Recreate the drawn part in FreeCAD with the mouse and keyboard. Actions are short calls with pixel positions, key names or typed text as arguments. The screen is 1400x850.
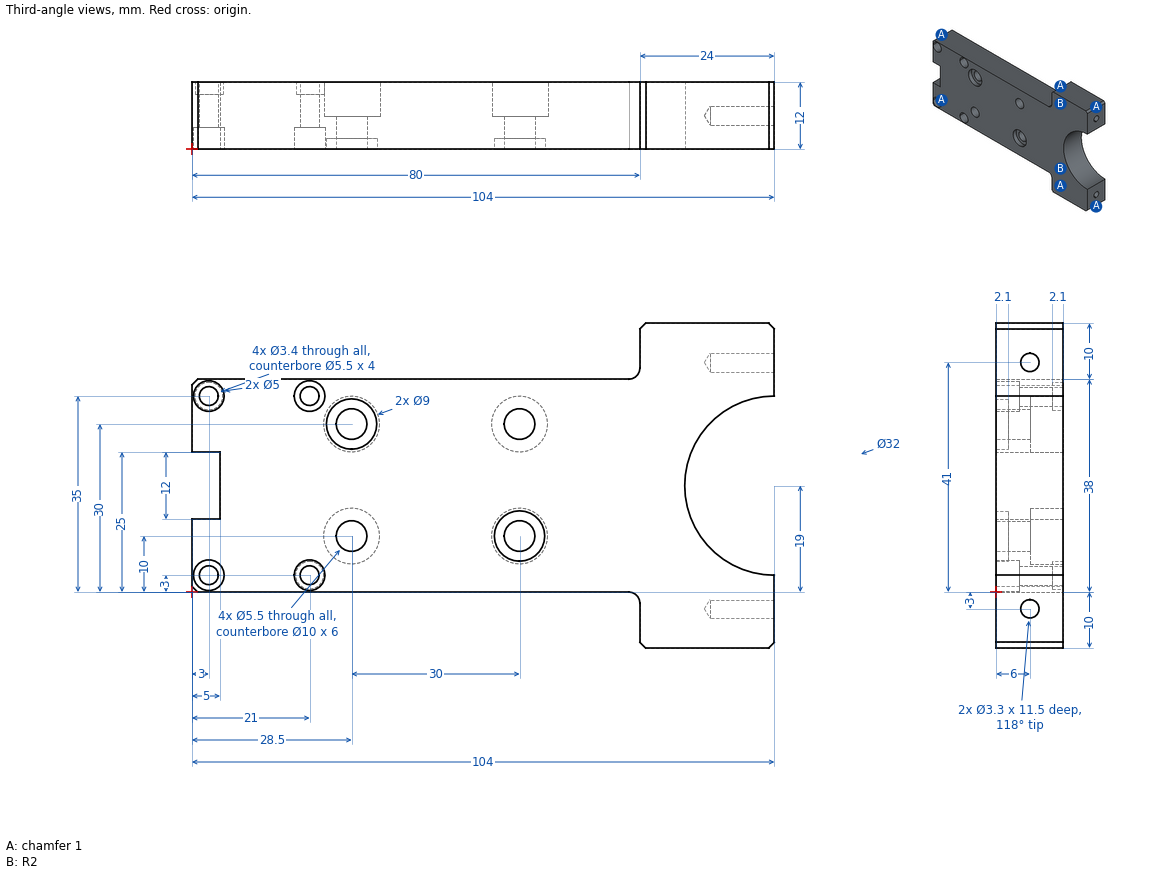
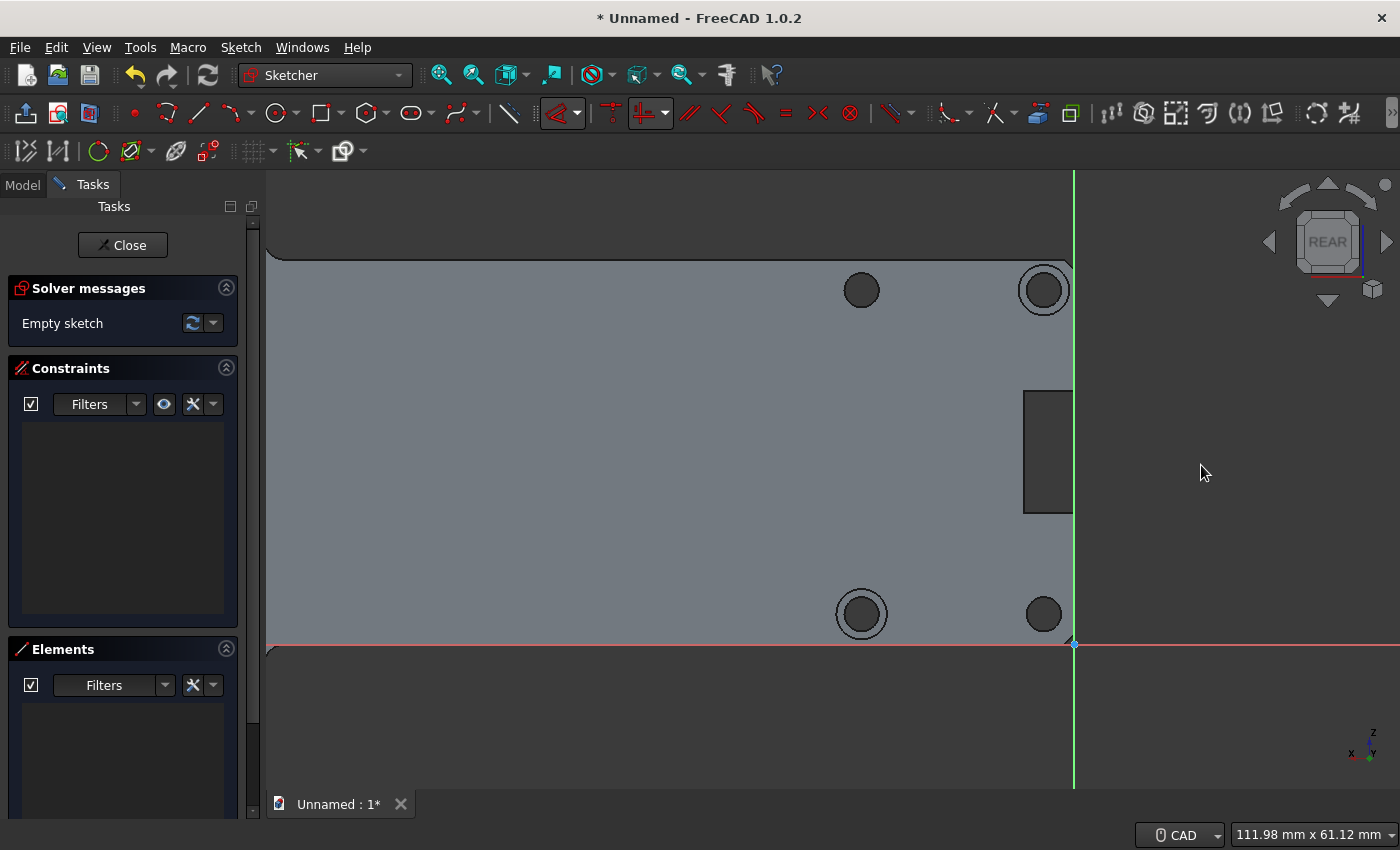
click(276, 114)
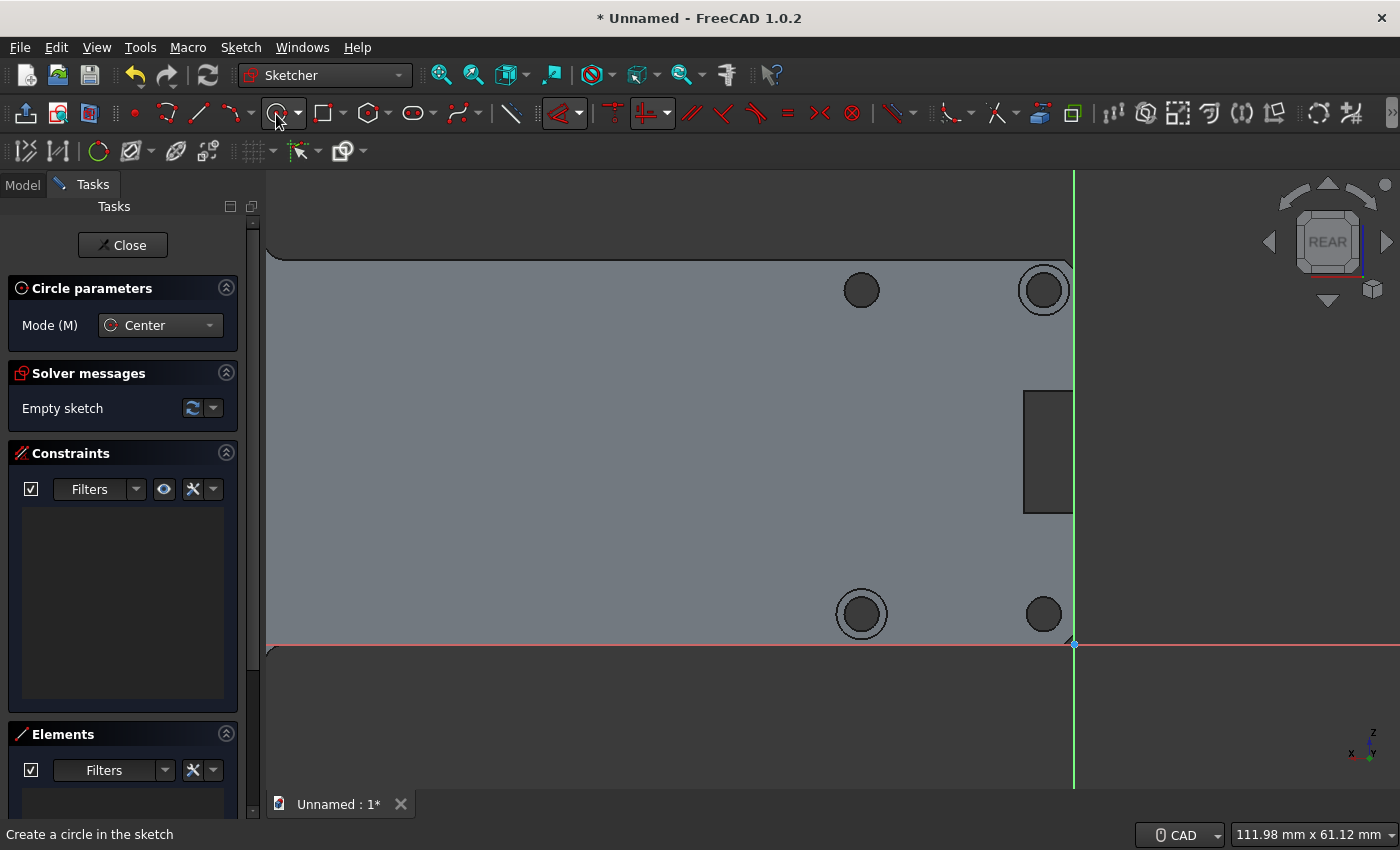
click(786, 543)
click(805, 524)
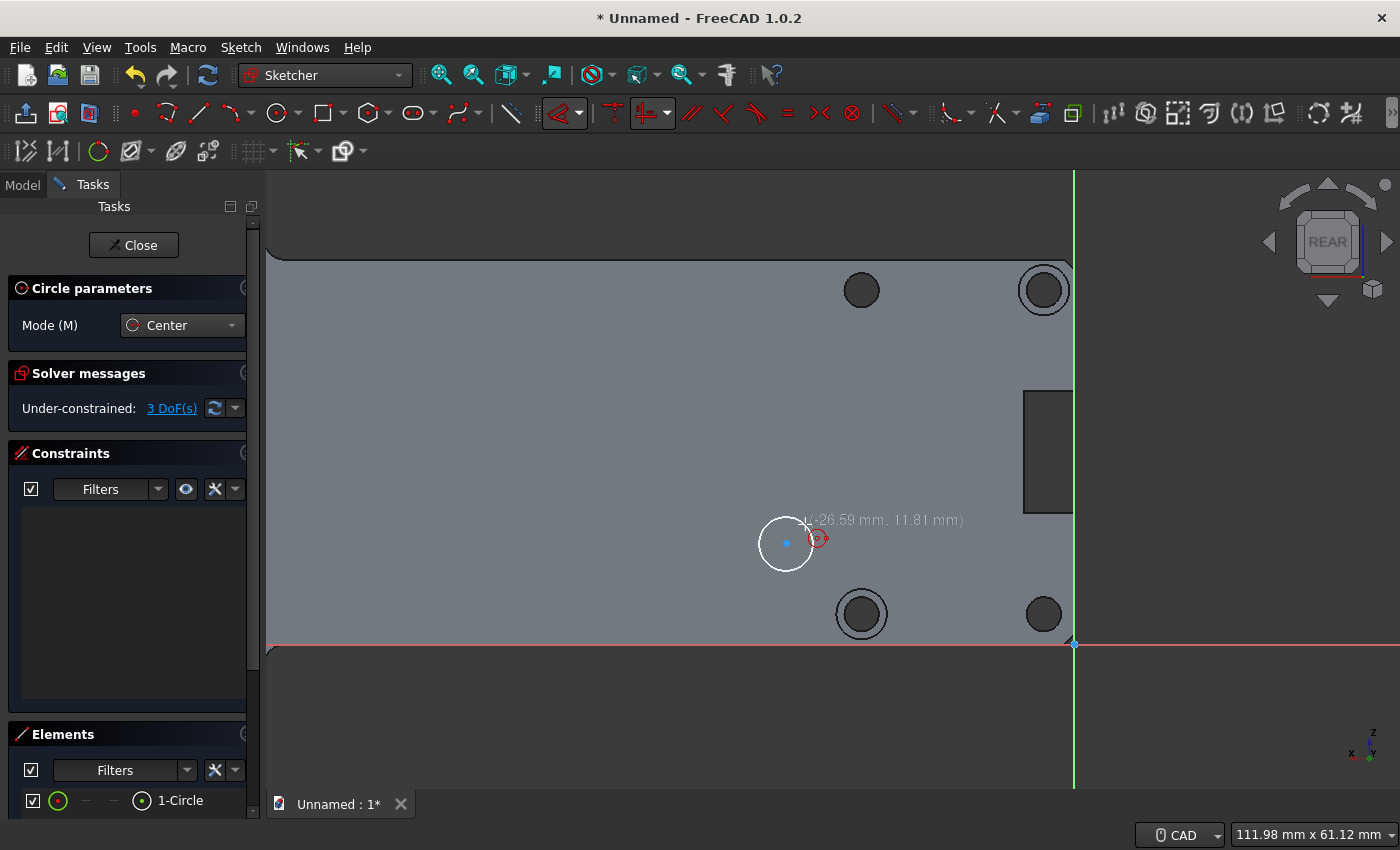
click(786, 341)
click(805, 321)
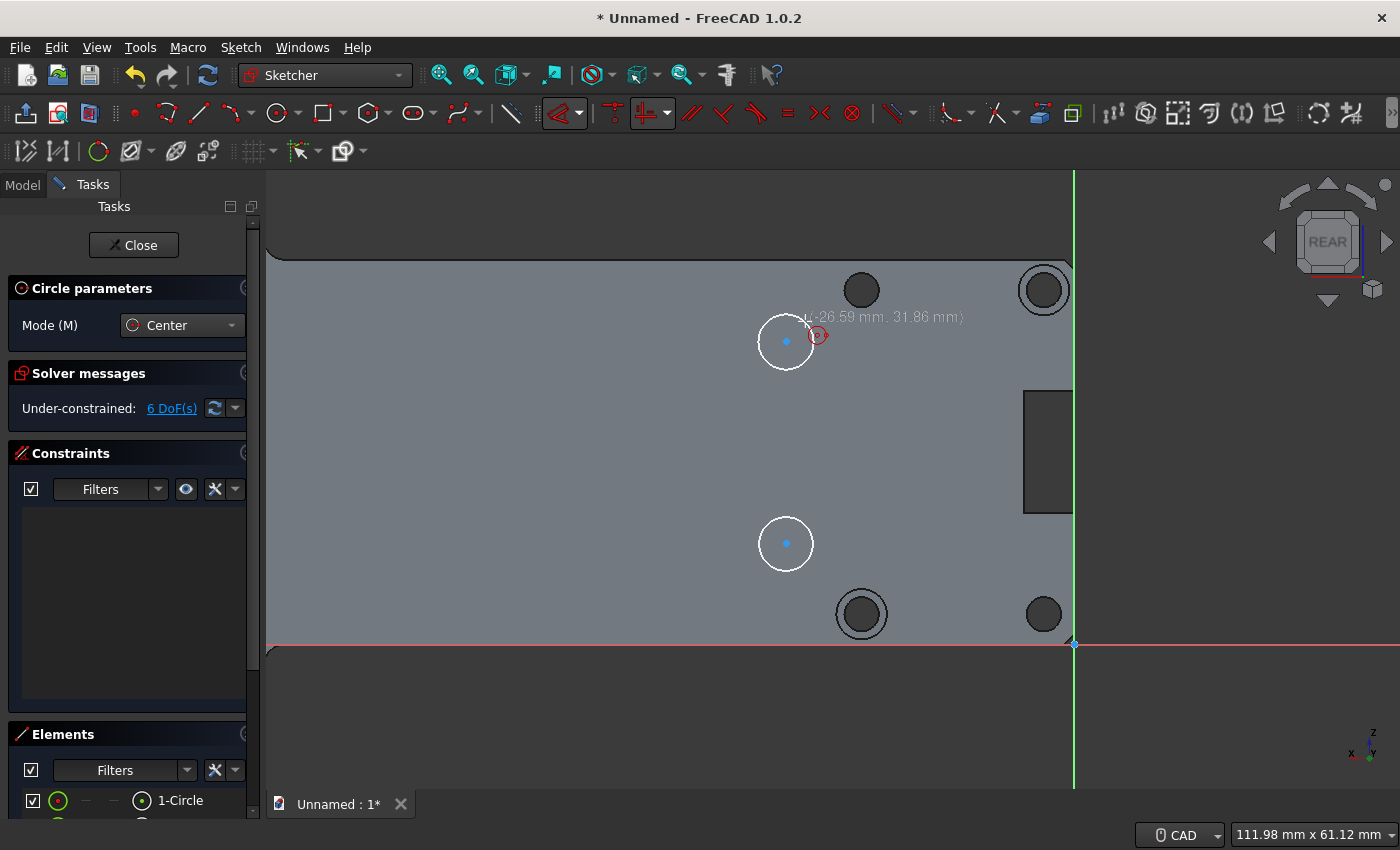
click(482, 543)
click(502, 524)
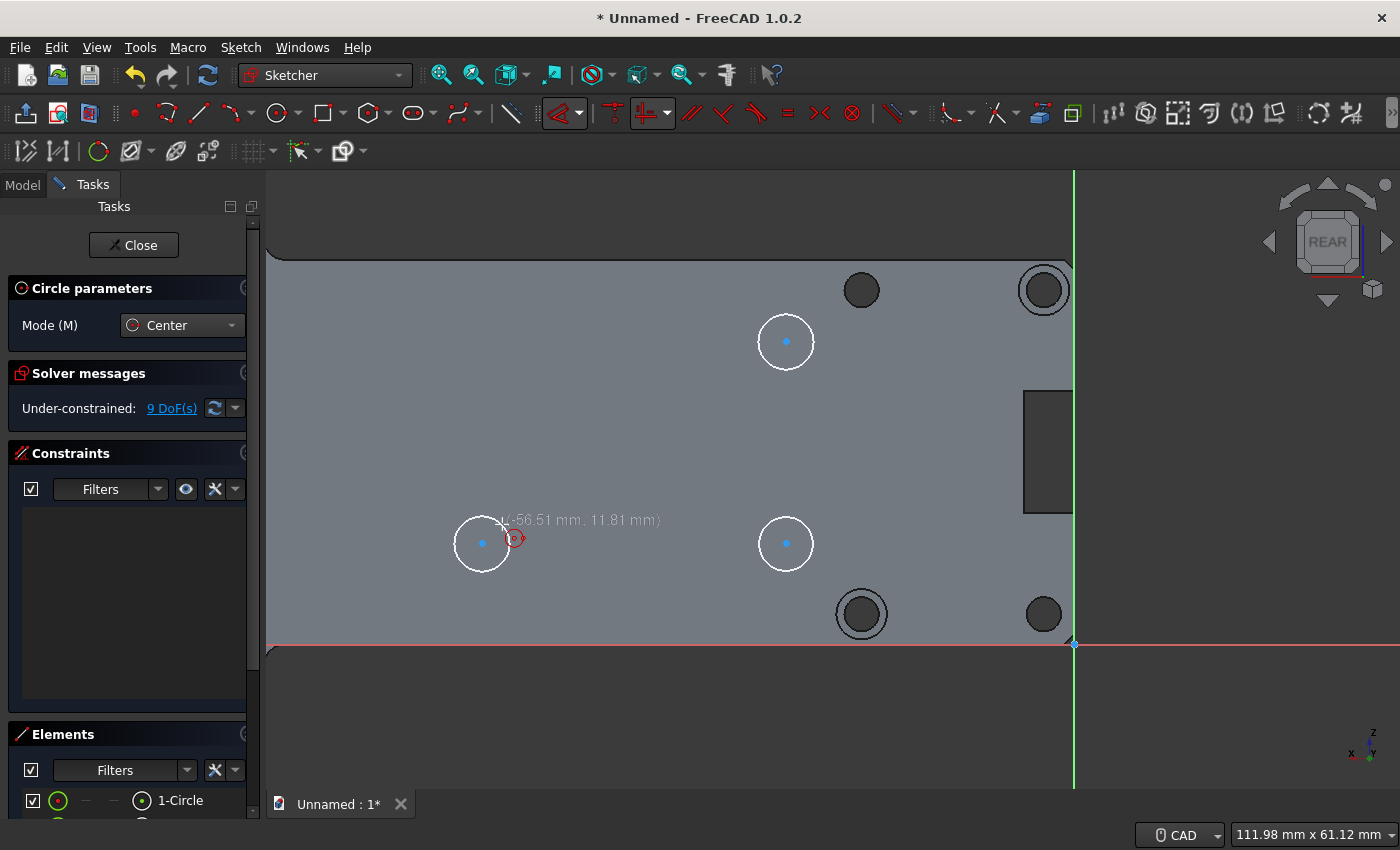
click(482, 341)
click(502, 321)
key(Escape)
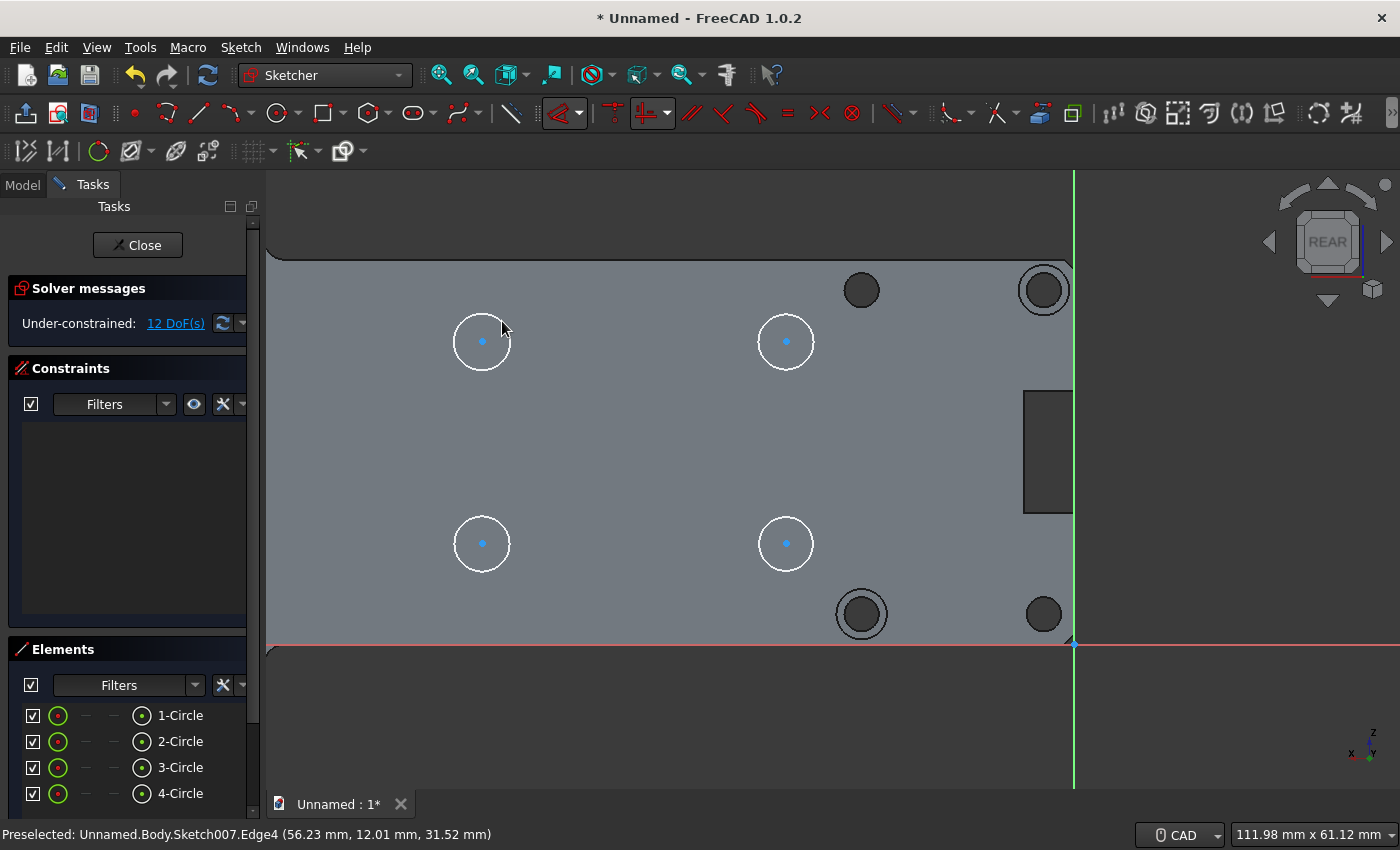
click(805, 525)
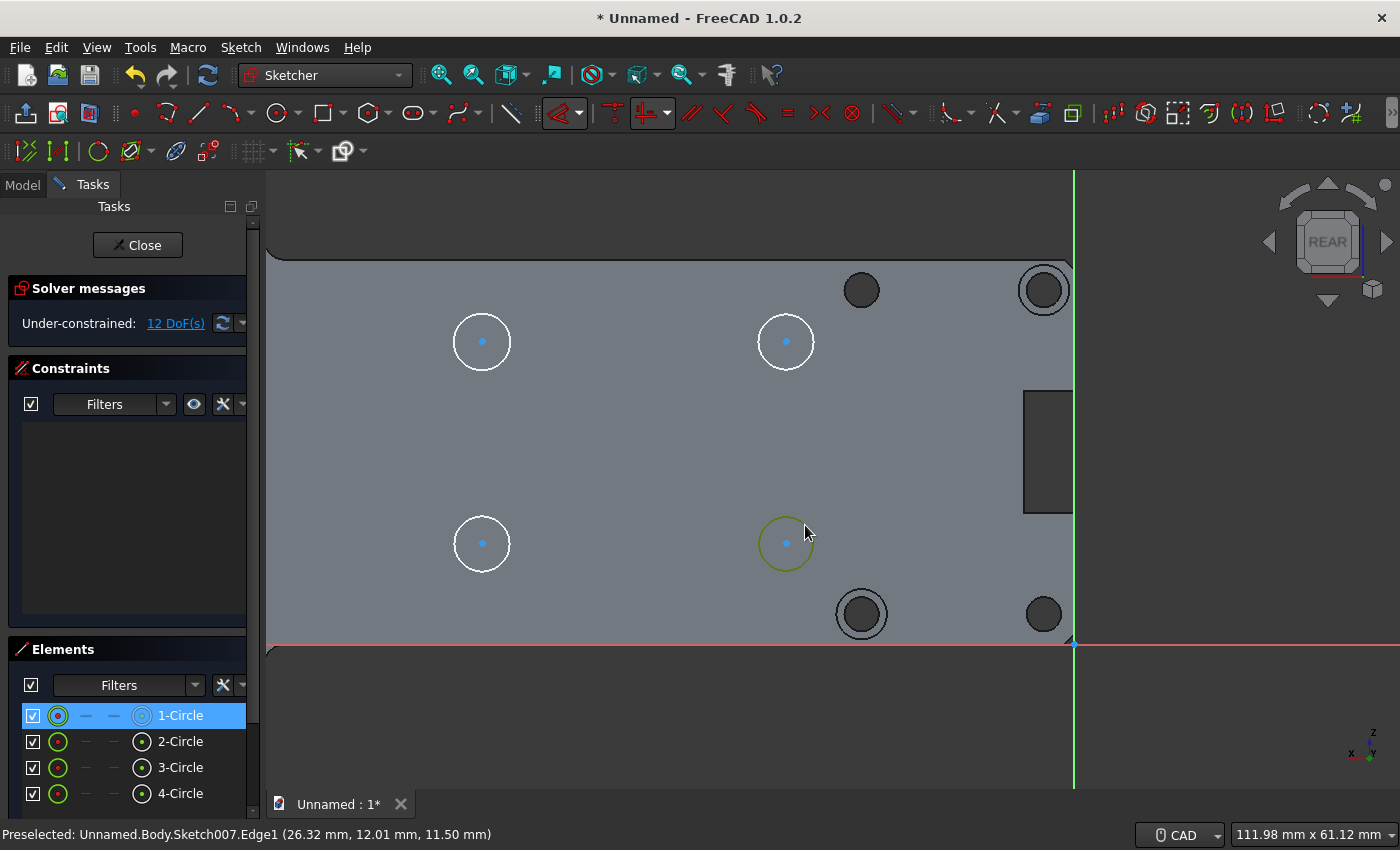
click(805, 322)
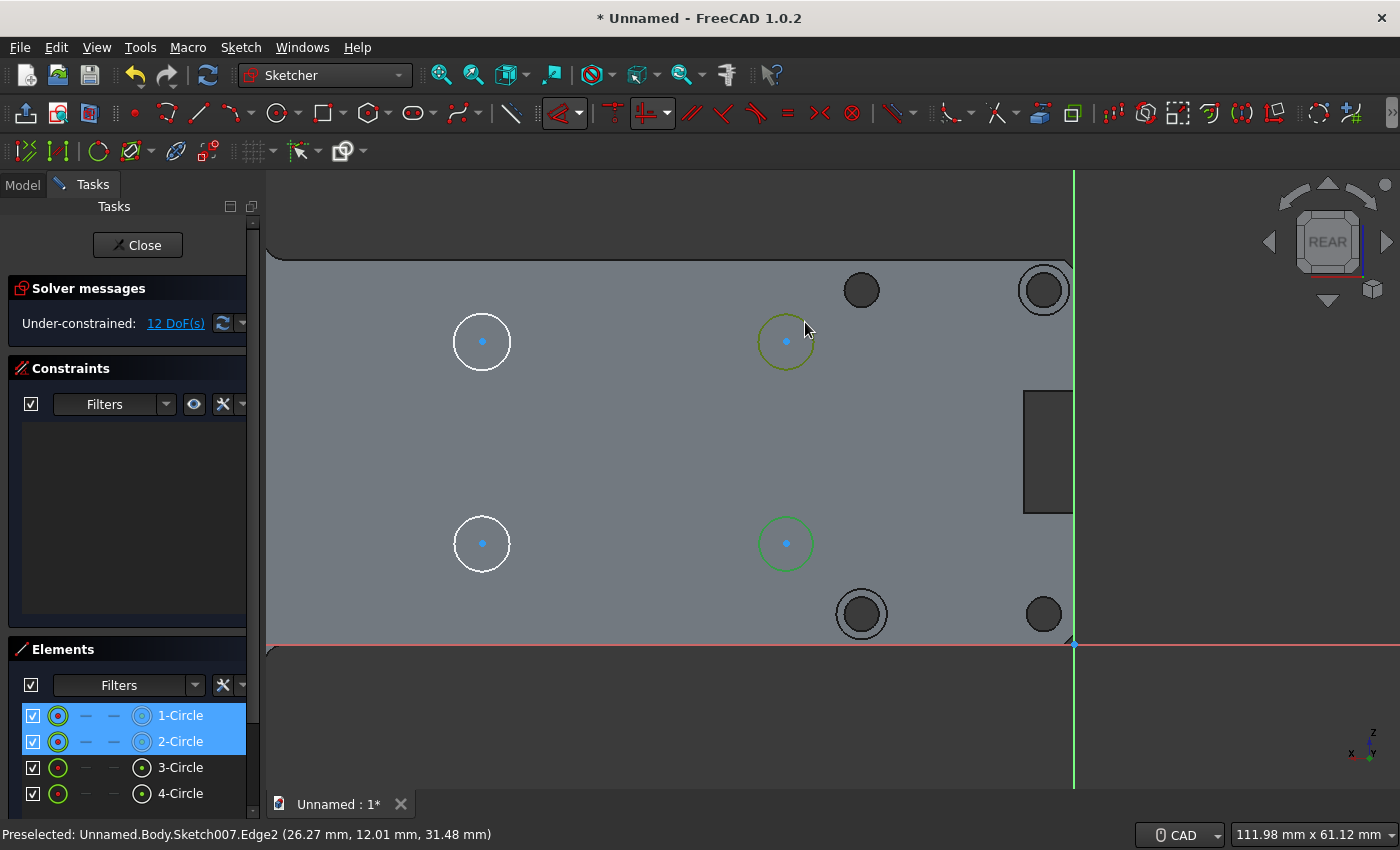
click(501, 524)